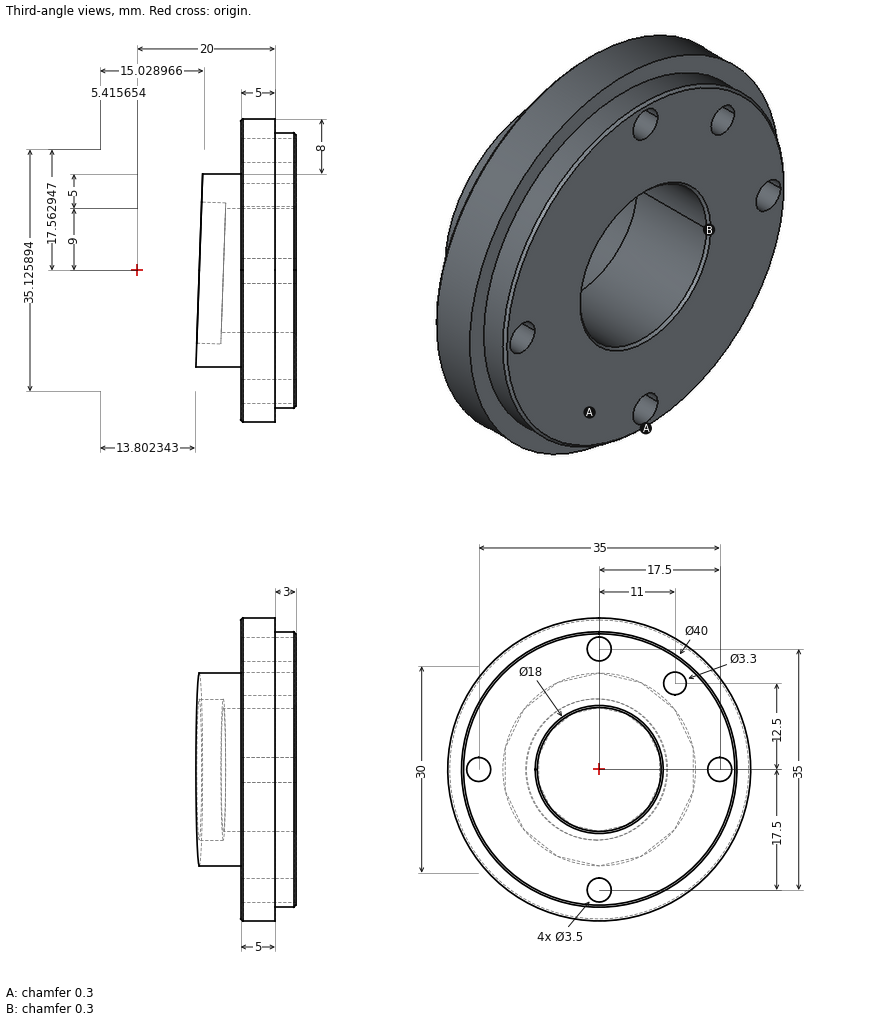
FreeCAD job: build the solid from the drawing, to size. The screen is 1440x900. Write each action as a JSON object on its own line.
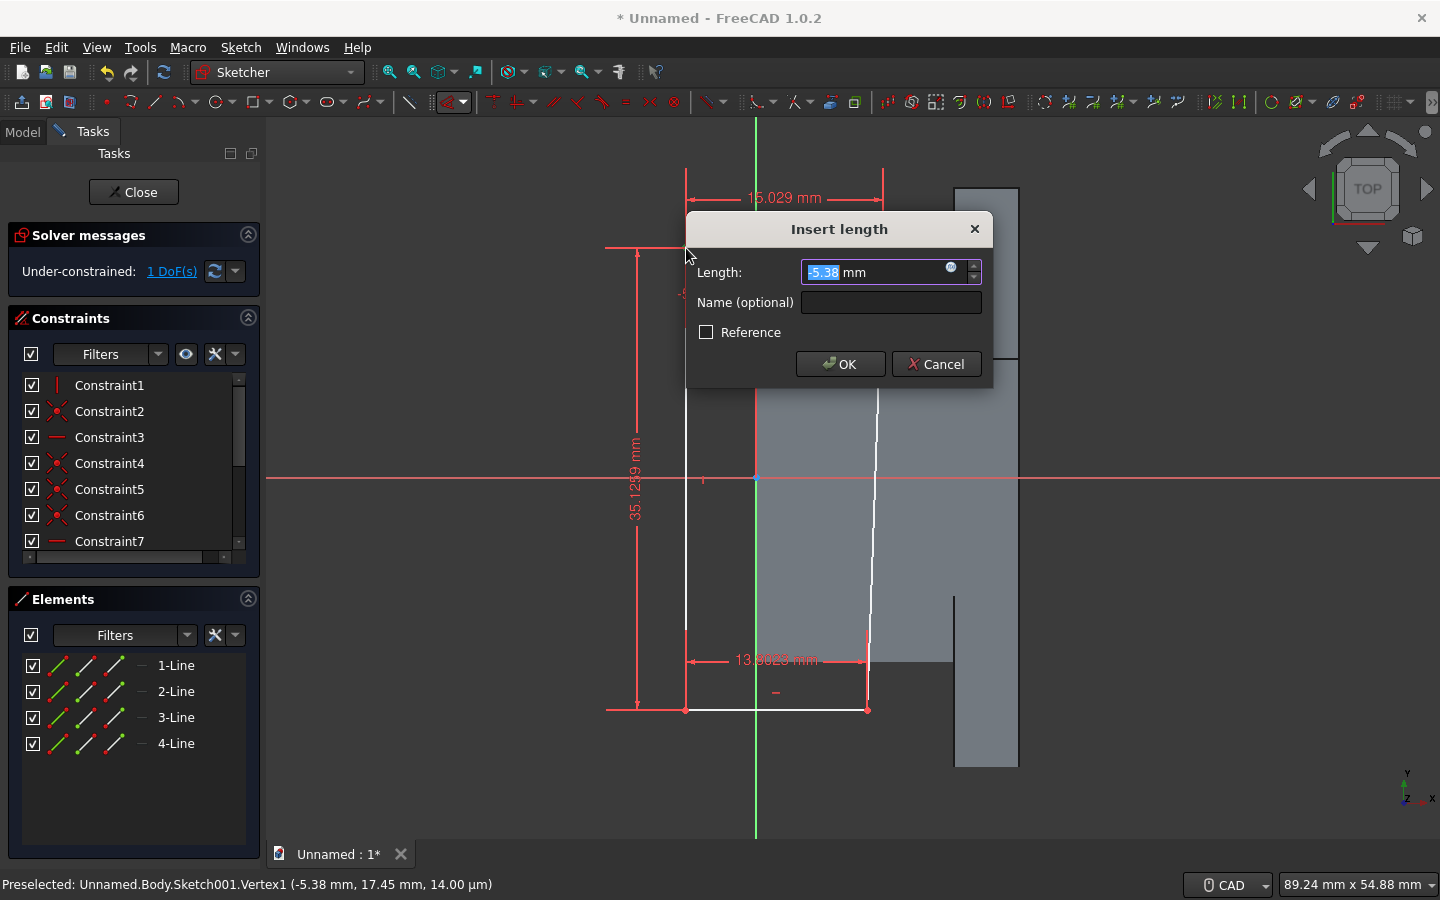
{"action": "type", "text": "-5.415654"}
{"action": "key", "text": "Return"}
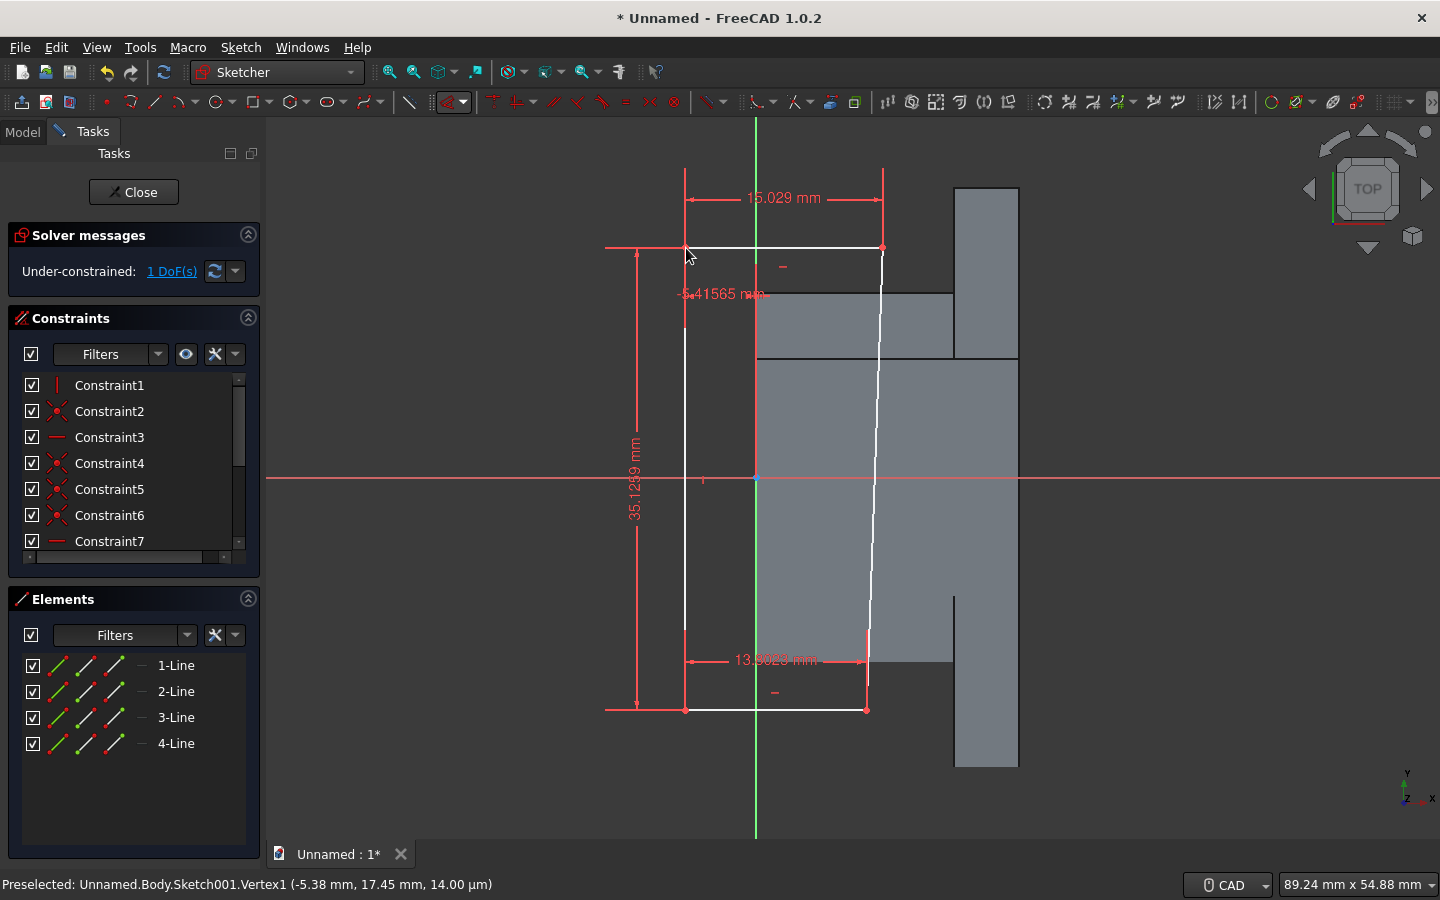
{"action": "left_click", "coordinate": [685, 248]}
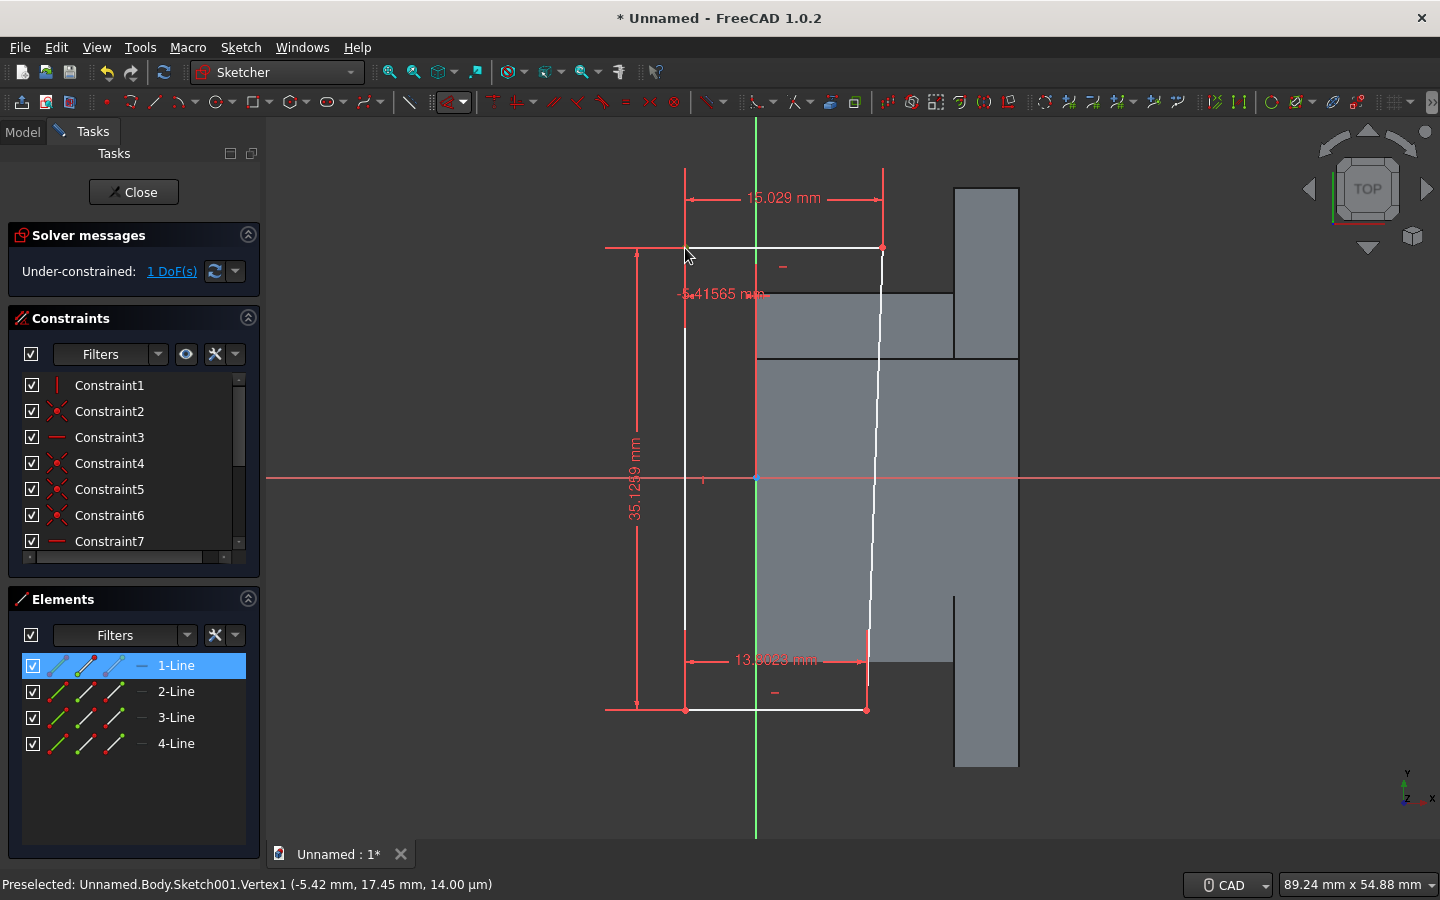
{"action": "left_click", "coordinate": [466, 102]}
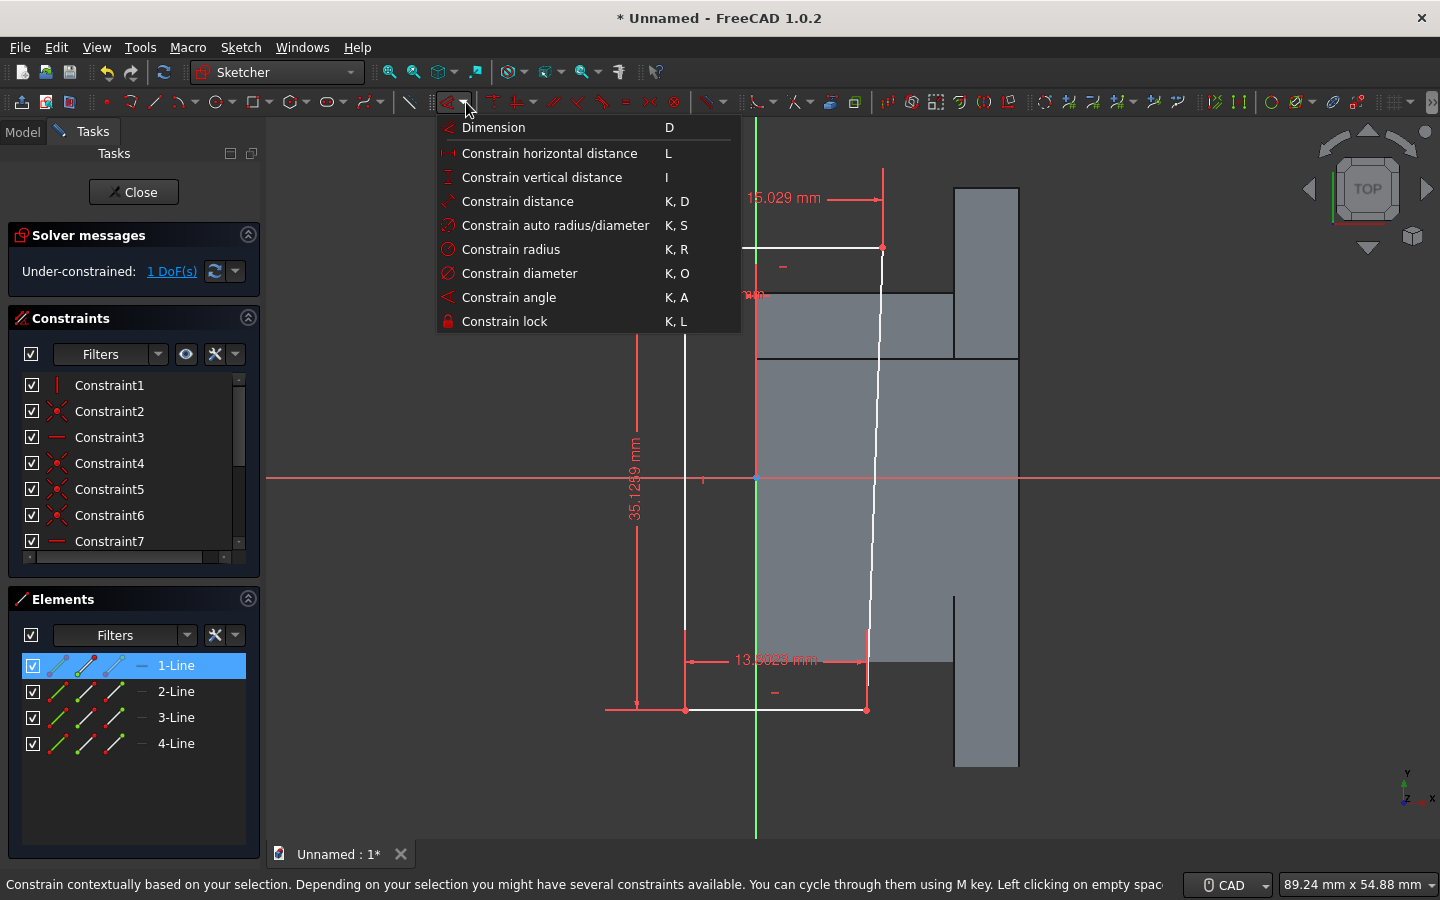
{"action": "left_click", "coordinate": [589, 177]}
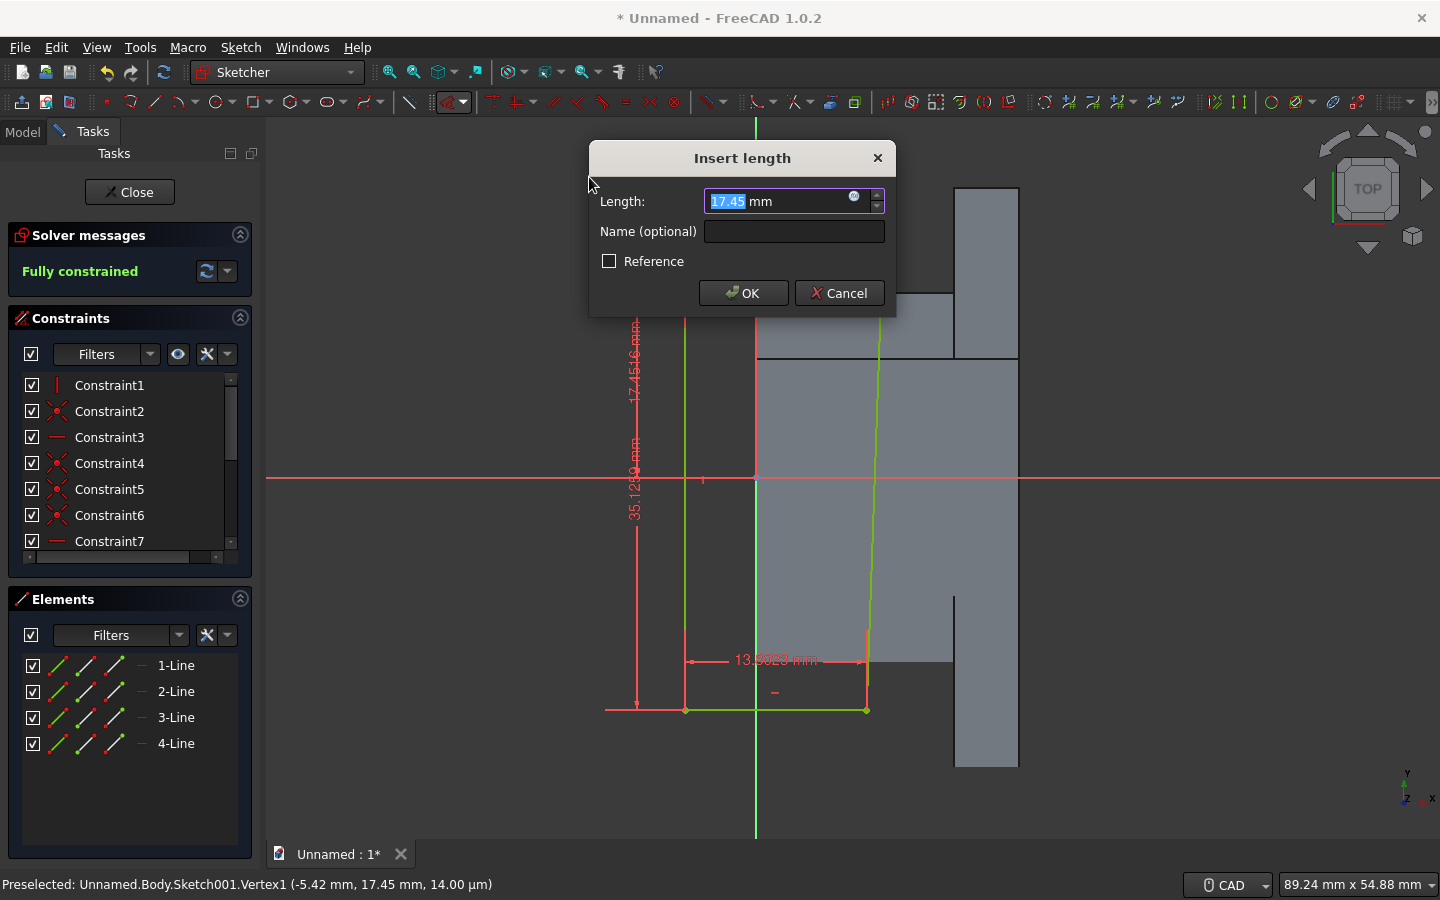
{"action": "type", "text": "17.562947"}
{"action": "key", "text": "Return"}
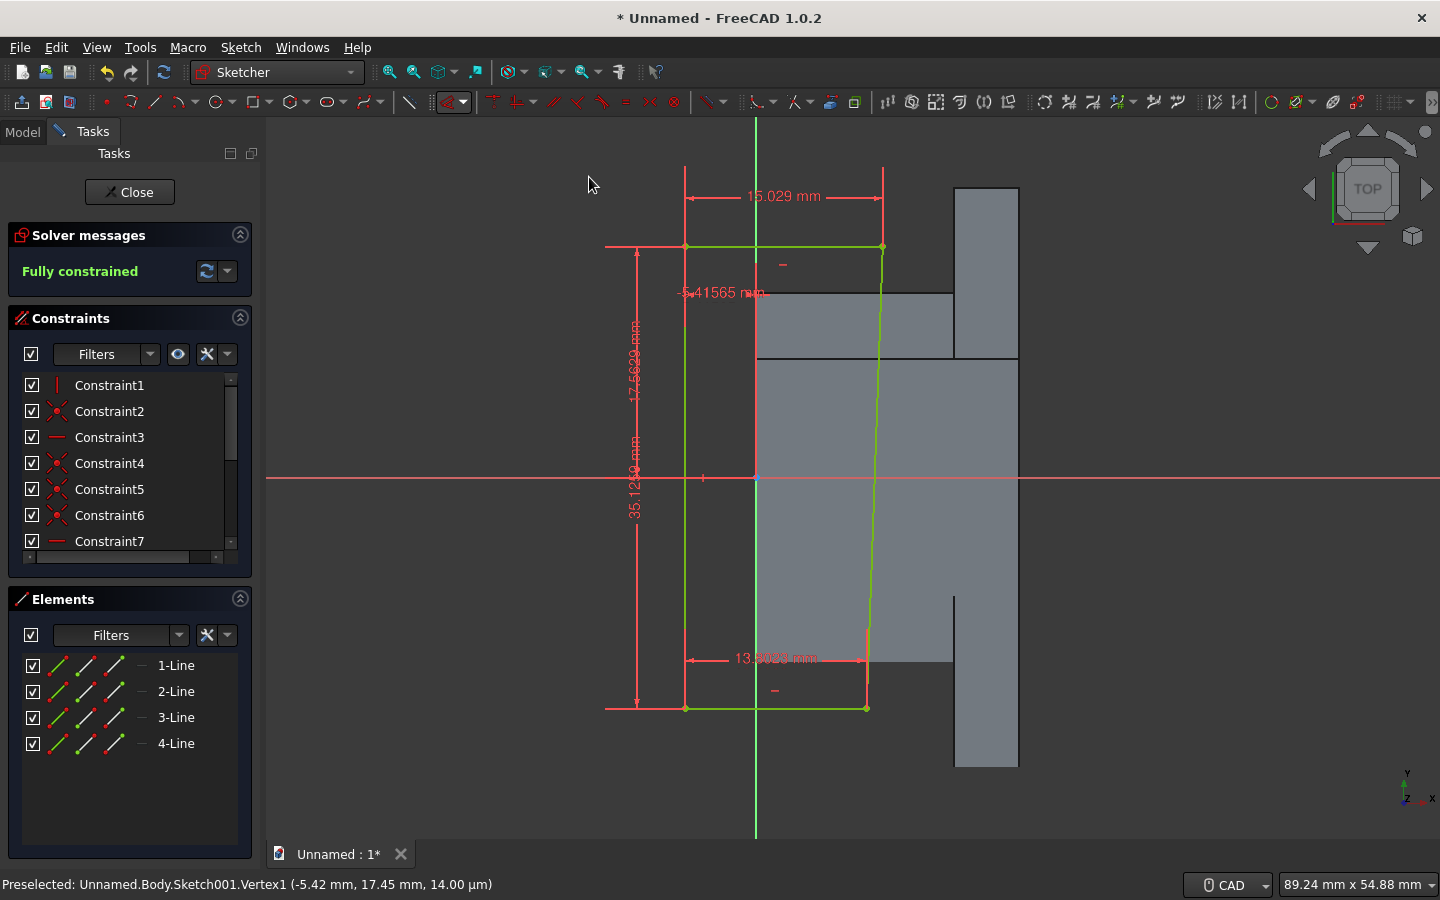
{"action": "left_click", "coordinate": [130, 192]}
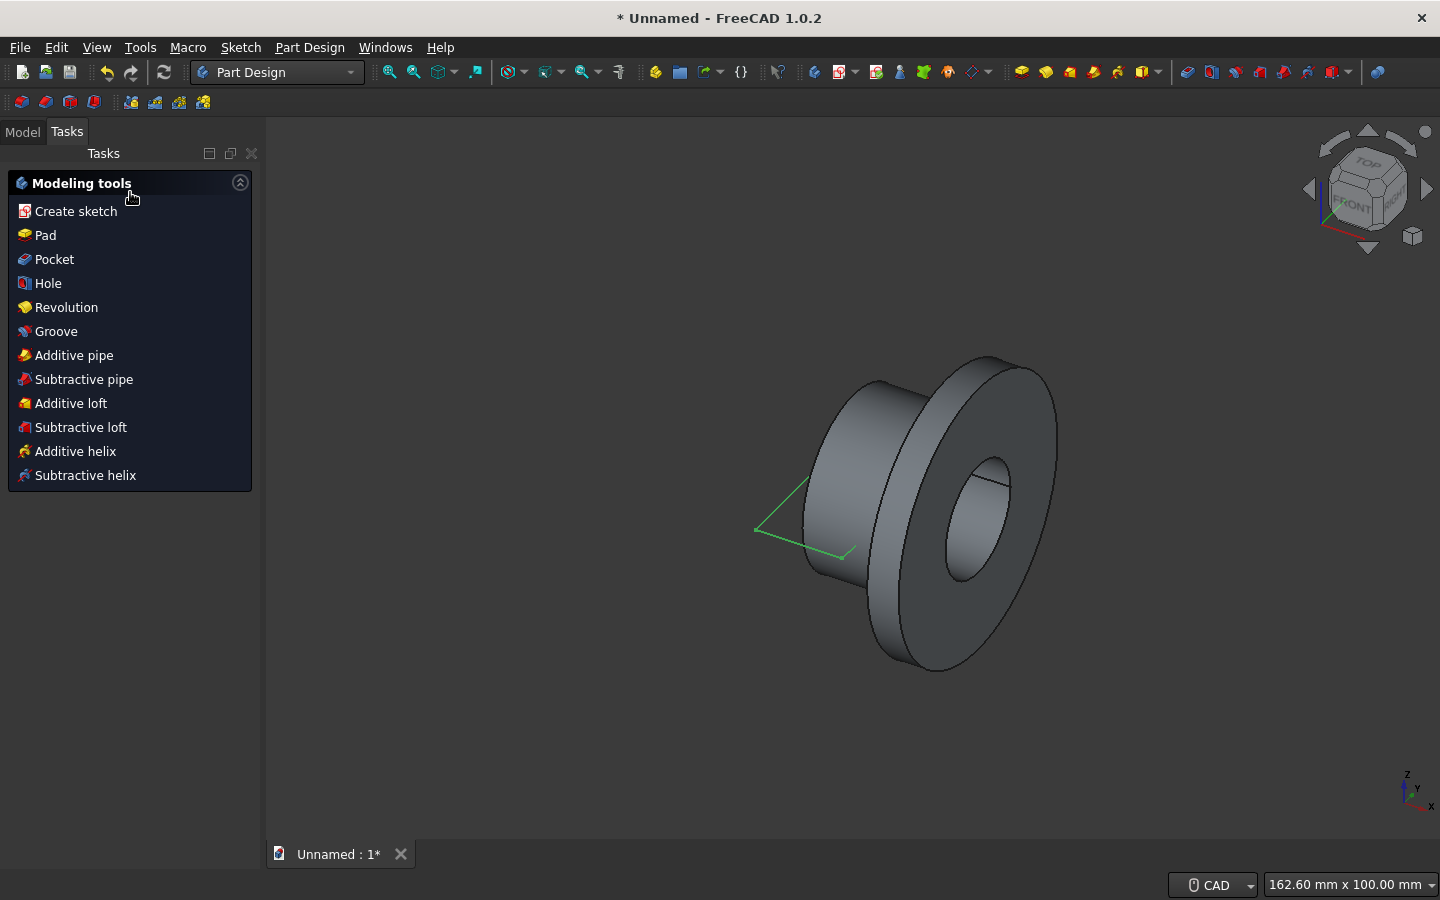
{"action": "left_click", "coordinate": [1188, 72]}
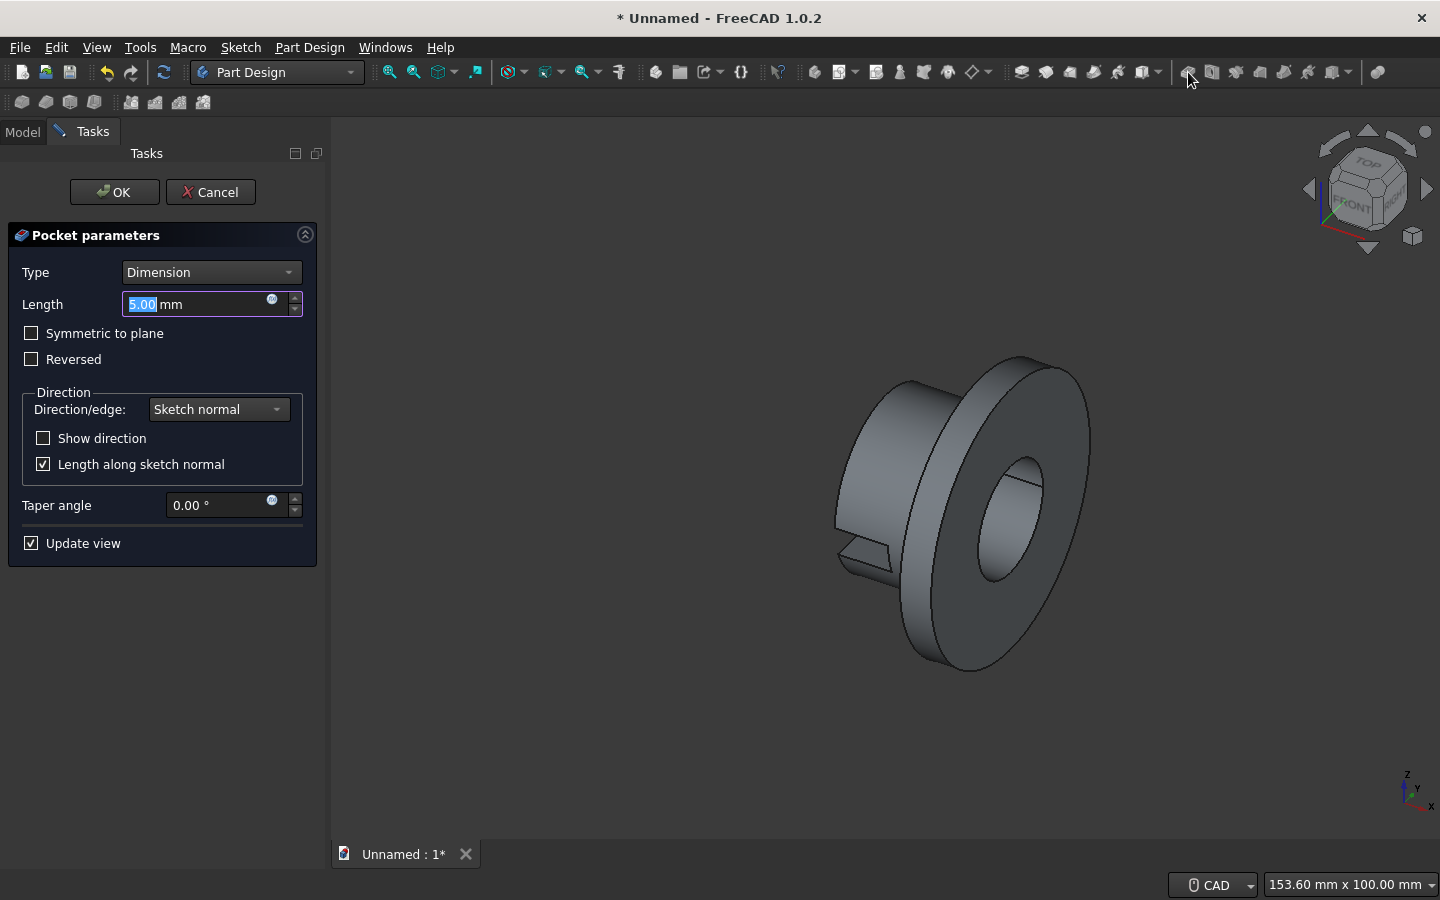
{"action": "type", "text": "30"}
{"action": "key", "text": "Tab"}